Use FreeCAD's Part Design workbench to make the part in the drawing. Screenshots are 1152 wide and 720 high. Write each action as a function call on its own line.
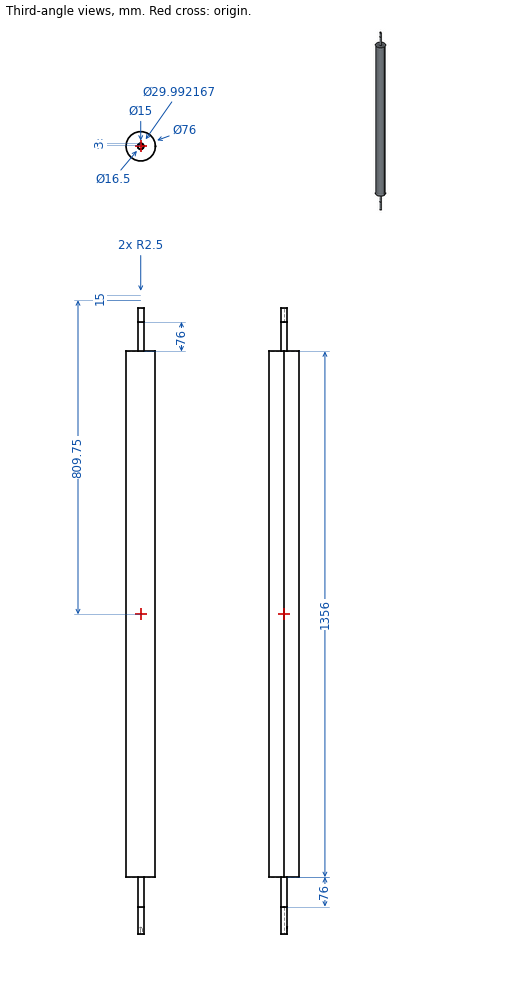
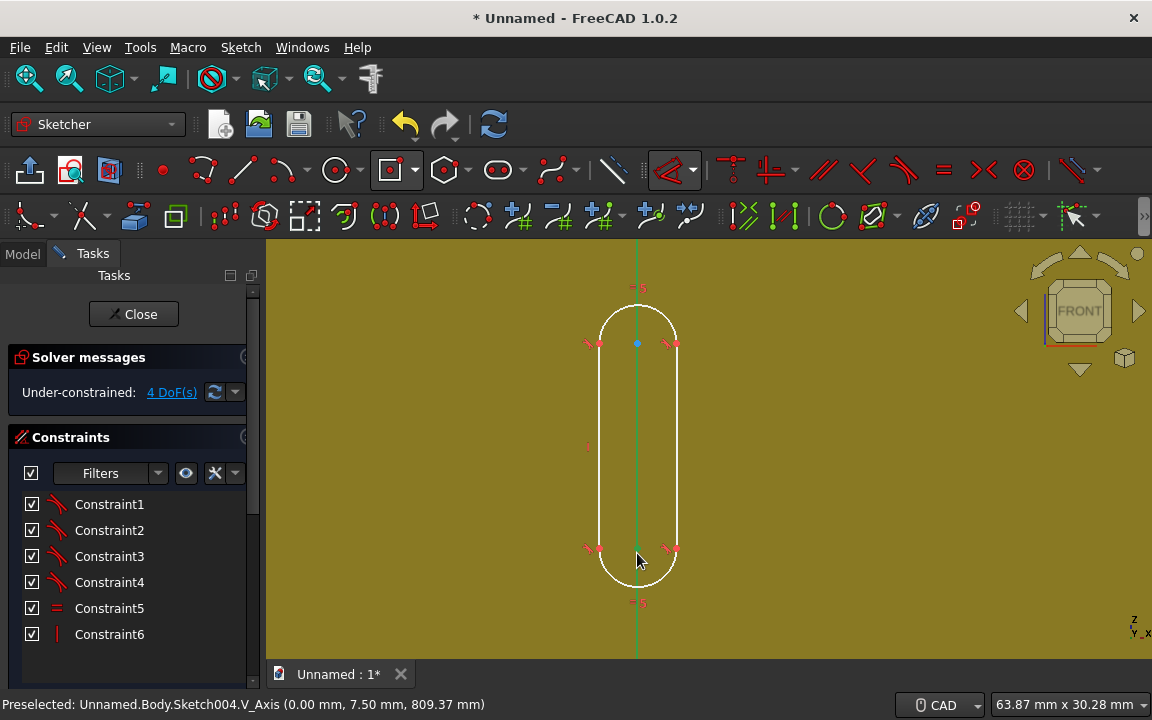
click(732, 170)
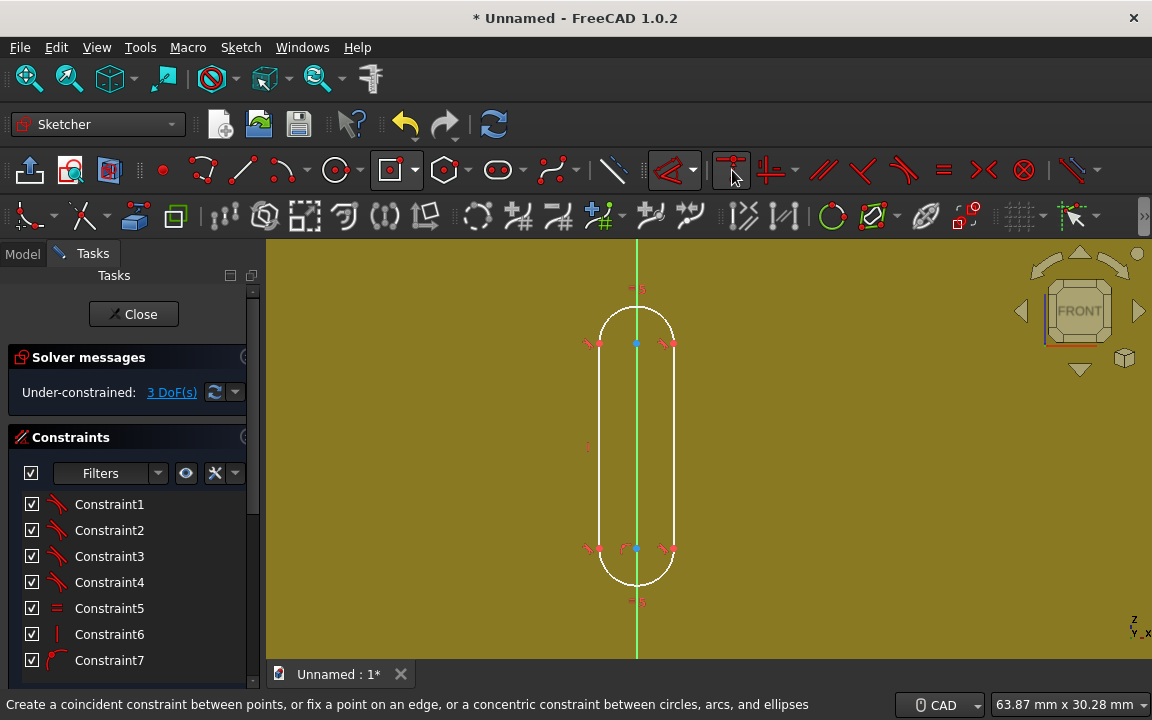
click(615, 579)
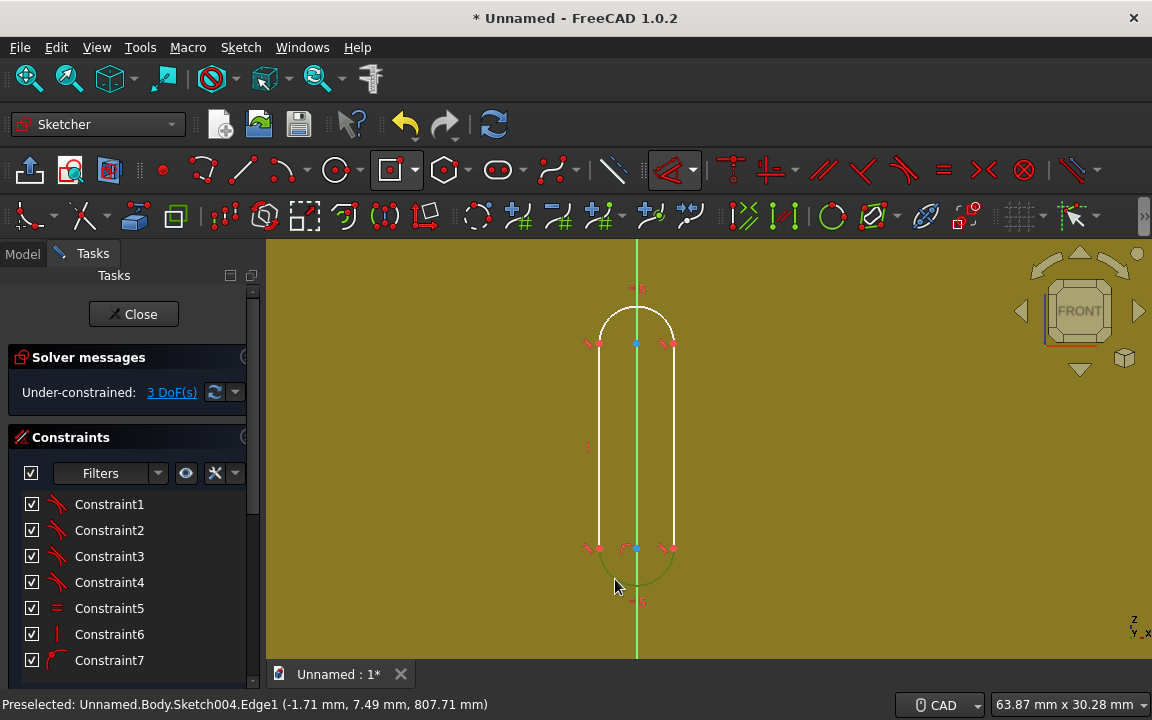
key(k)
key(r)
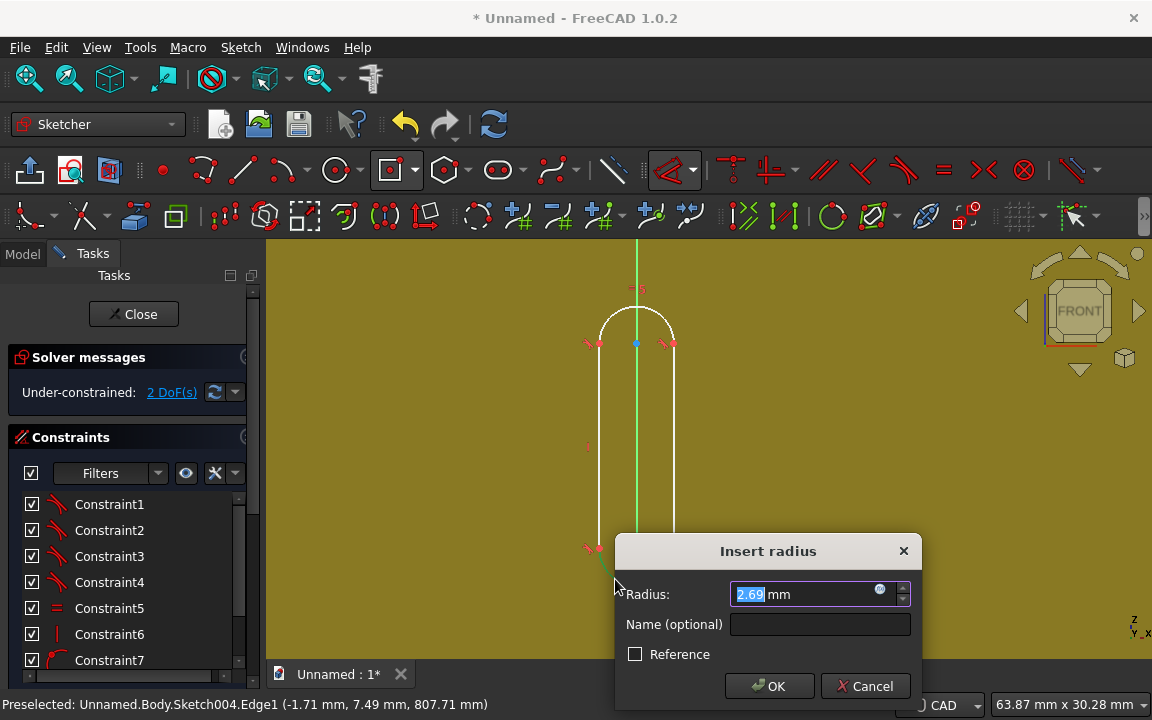
text(2.5)
key(Return)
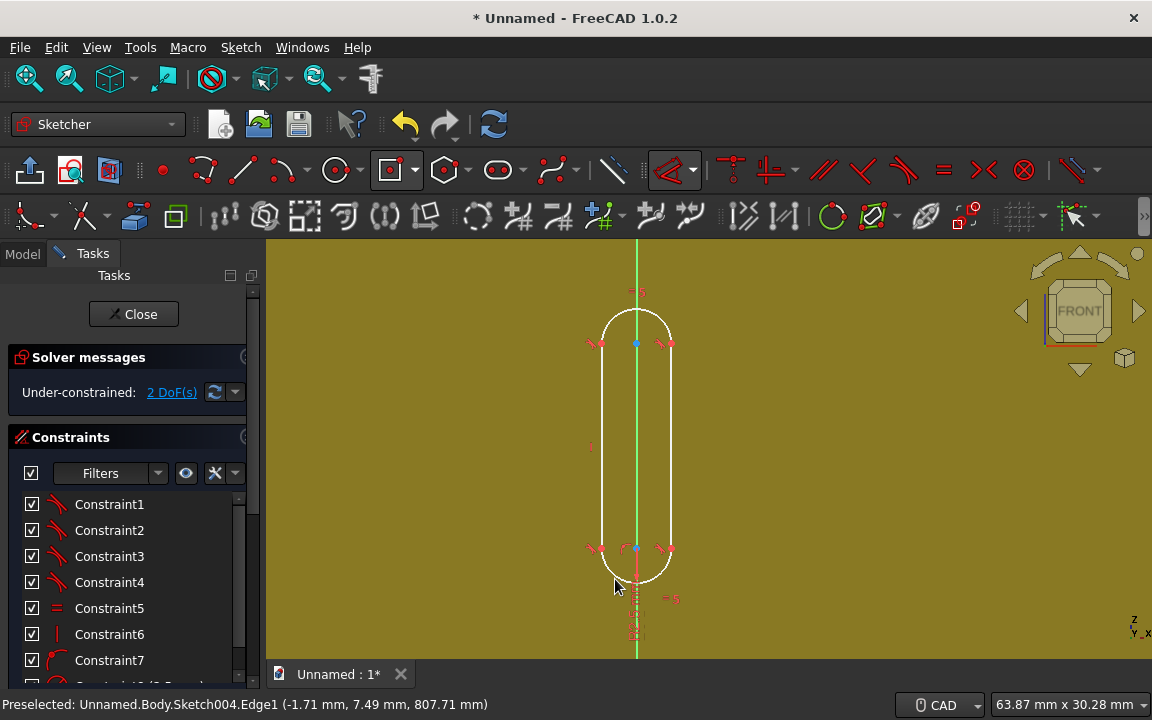
click(602, 487)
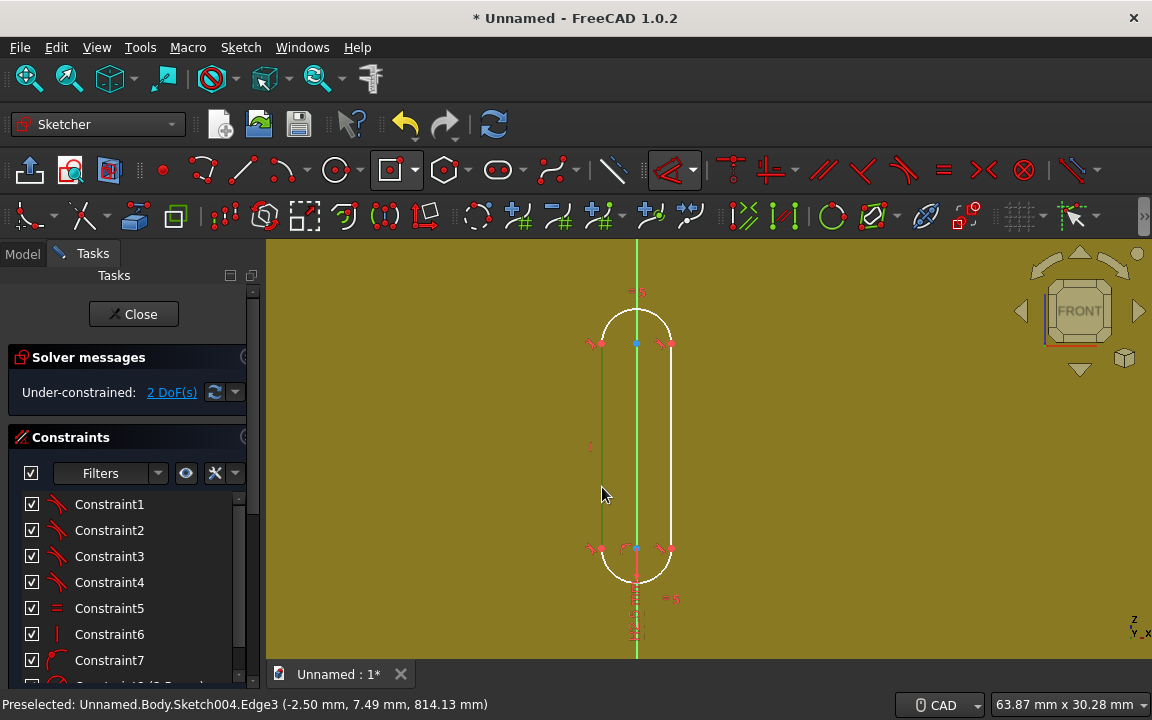
click(696, 170)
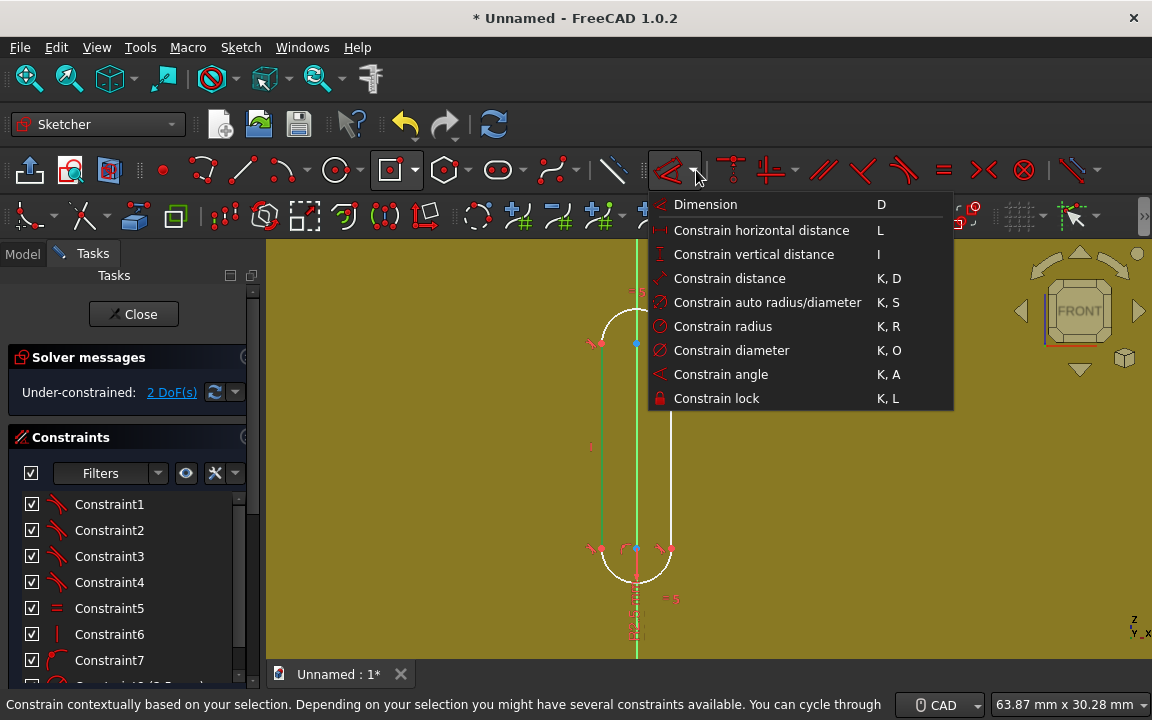
click(801, 254)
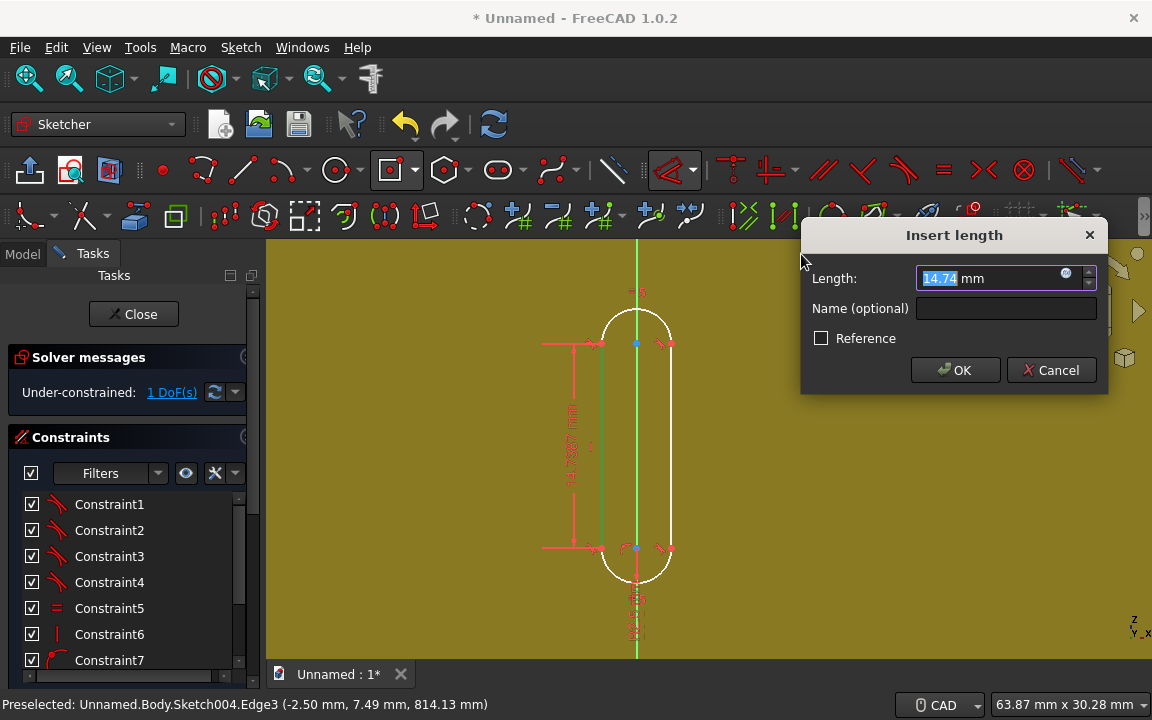
text(15)
key(Return)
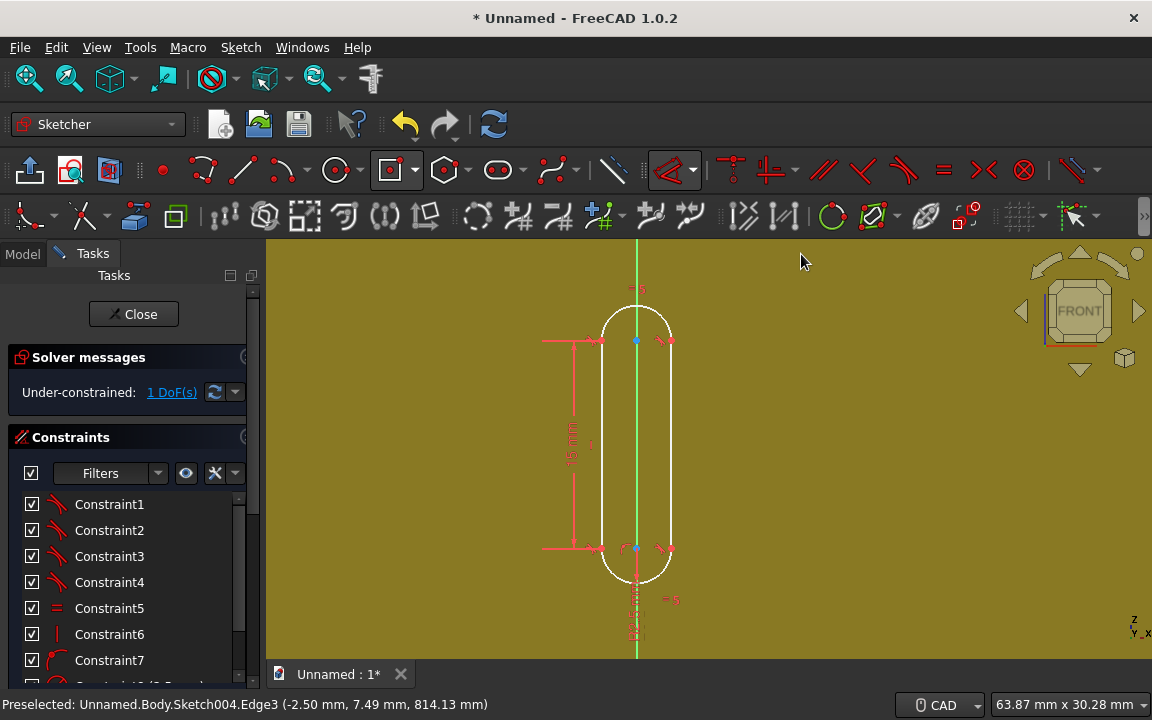
click(602, 549)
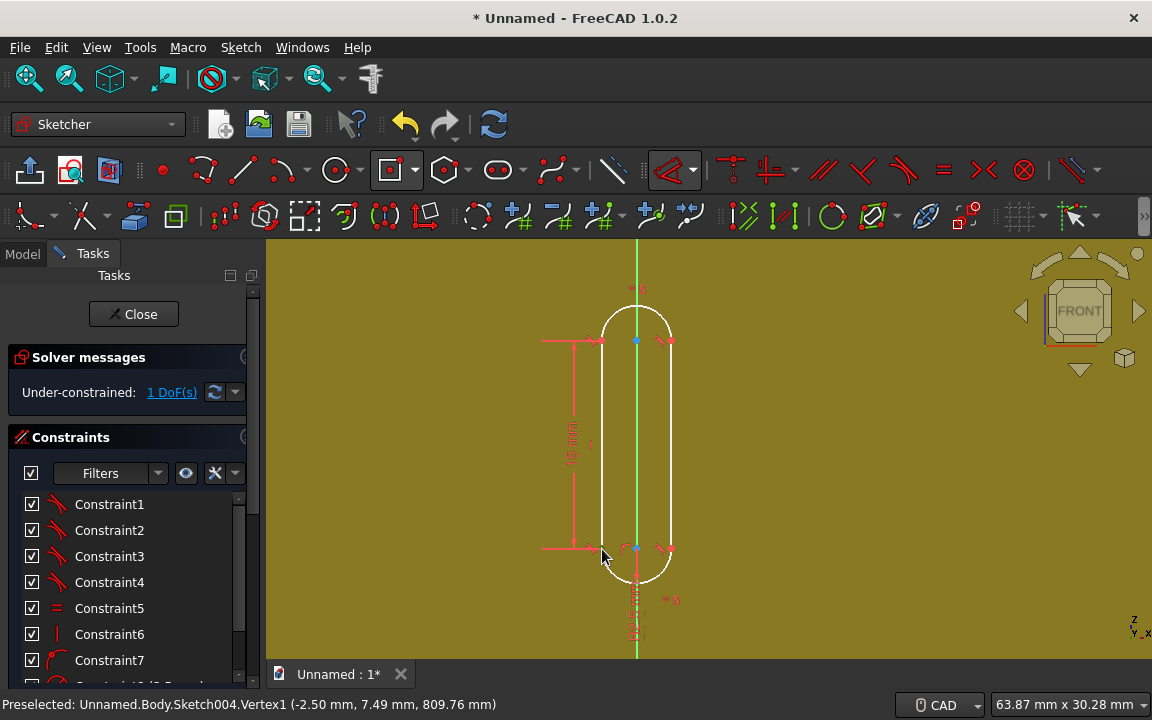
key(i)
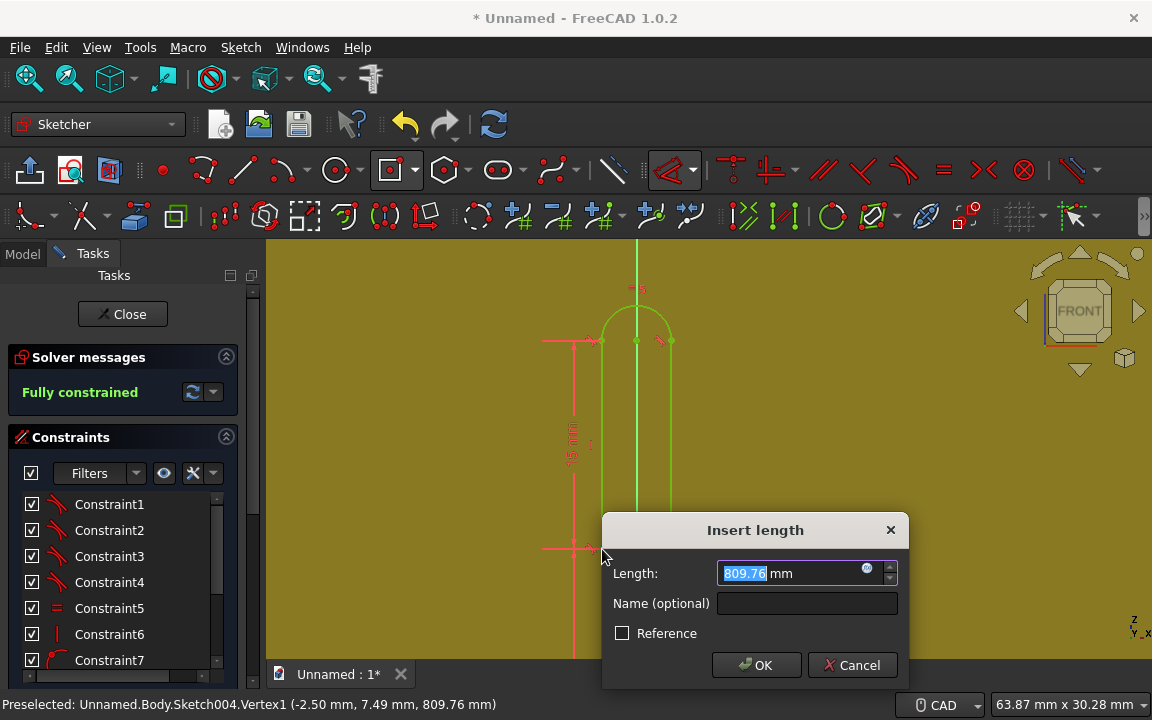
text(809.75)
key(Return)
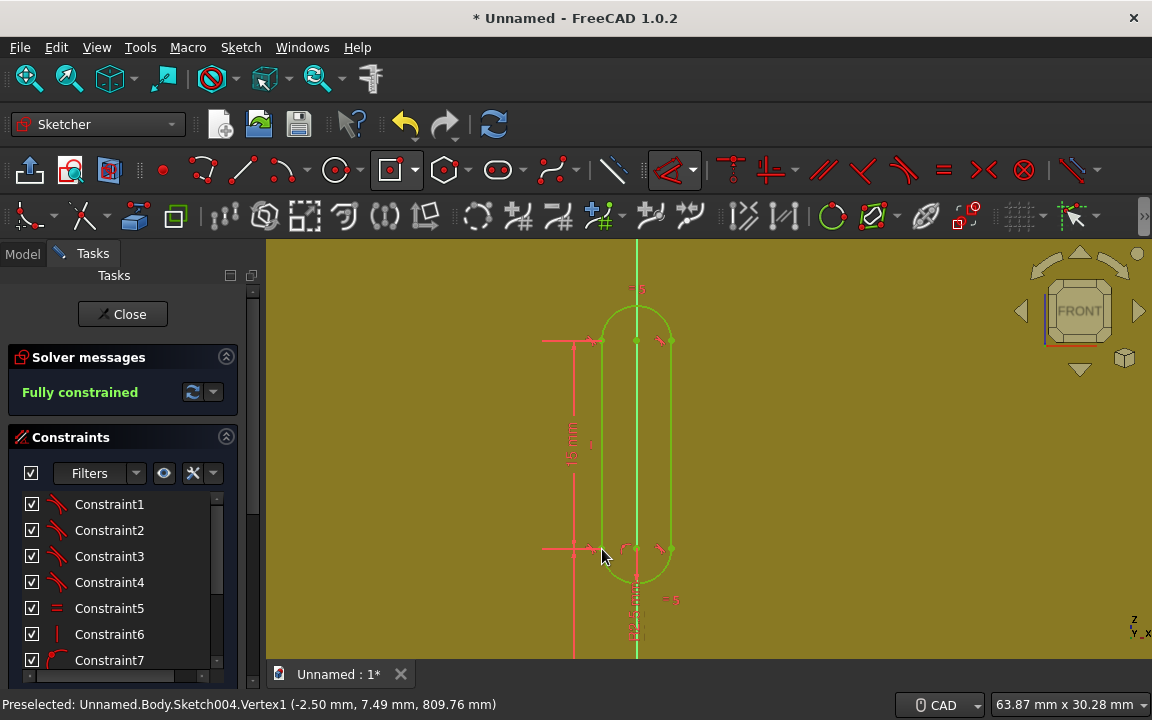
click(123, 314)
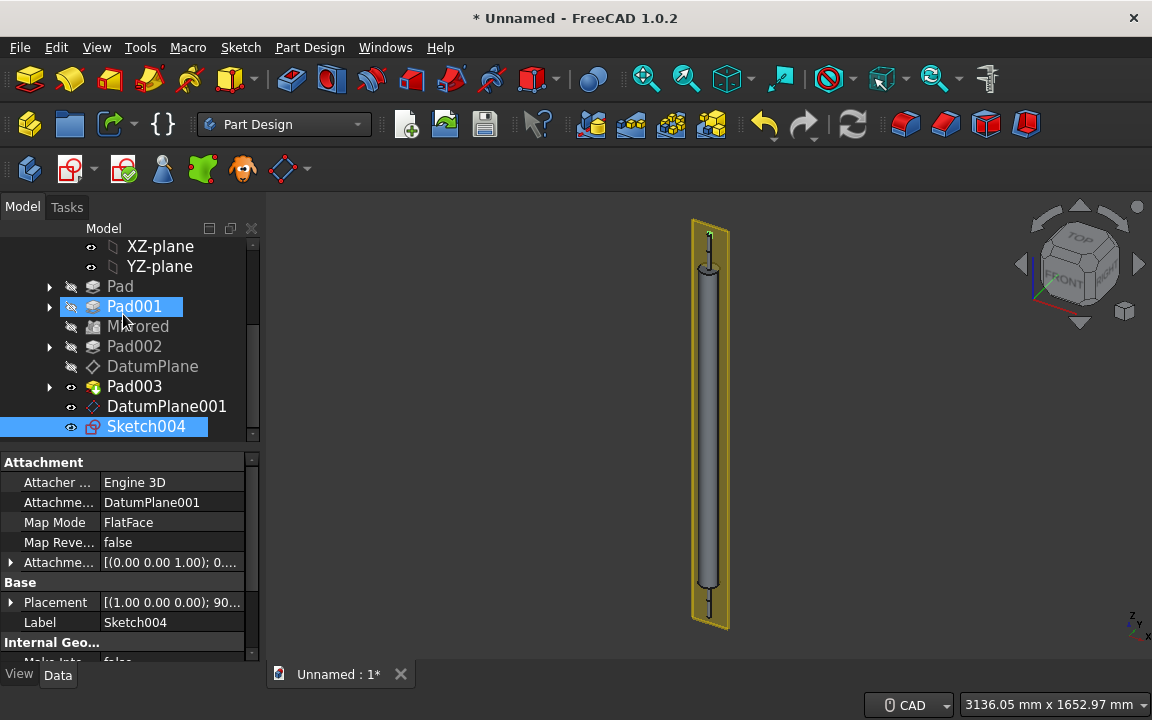
click(292, 80)